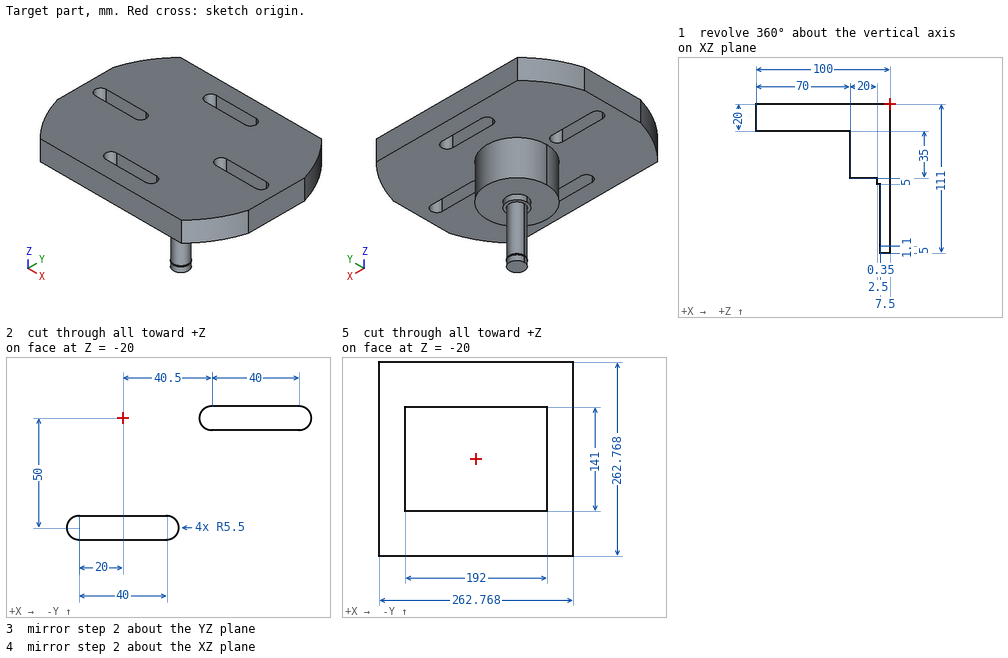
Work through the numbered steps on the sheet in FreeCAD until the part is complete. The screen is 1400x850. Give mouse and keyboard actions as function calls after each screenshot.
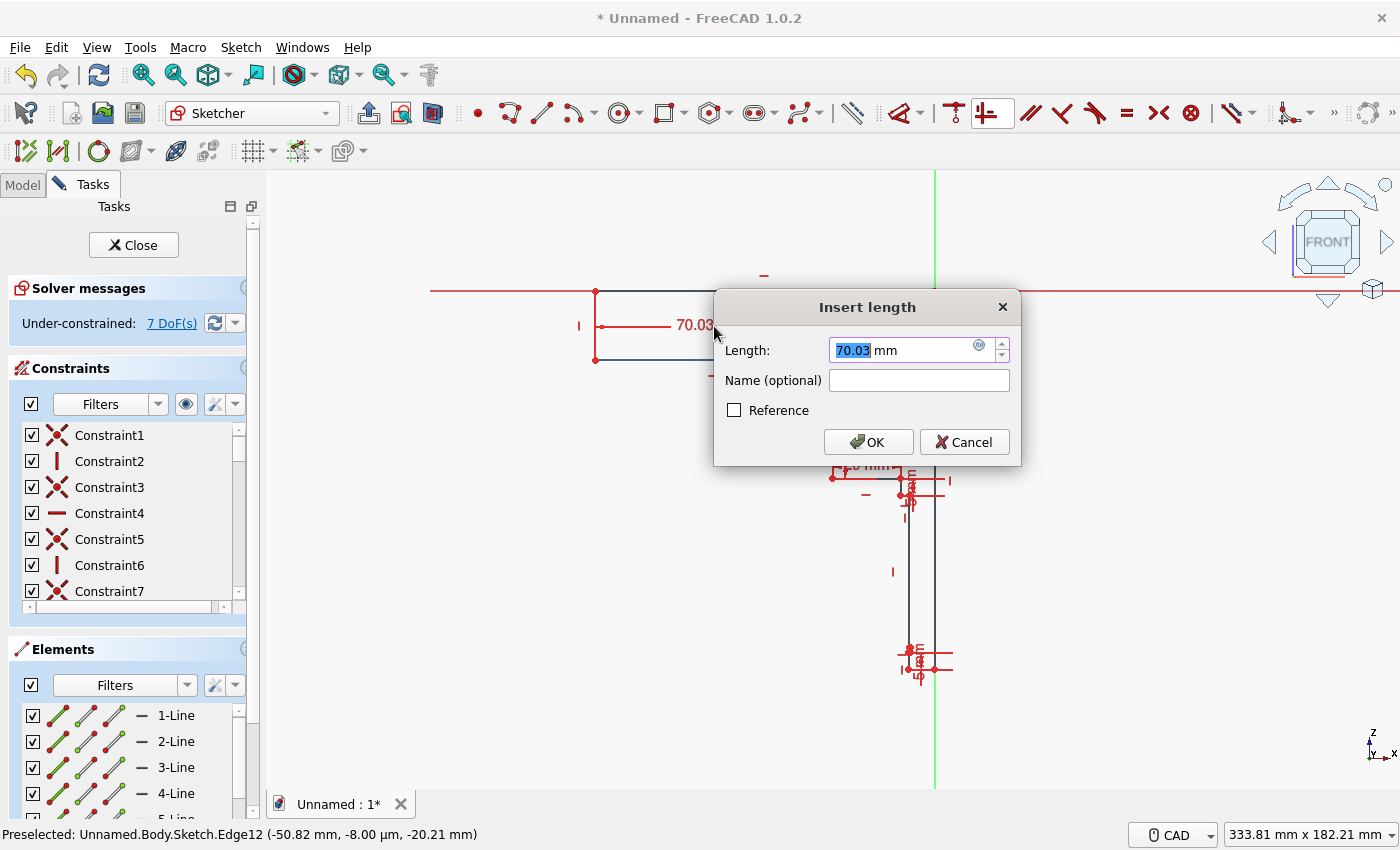
text(70)
key(Return)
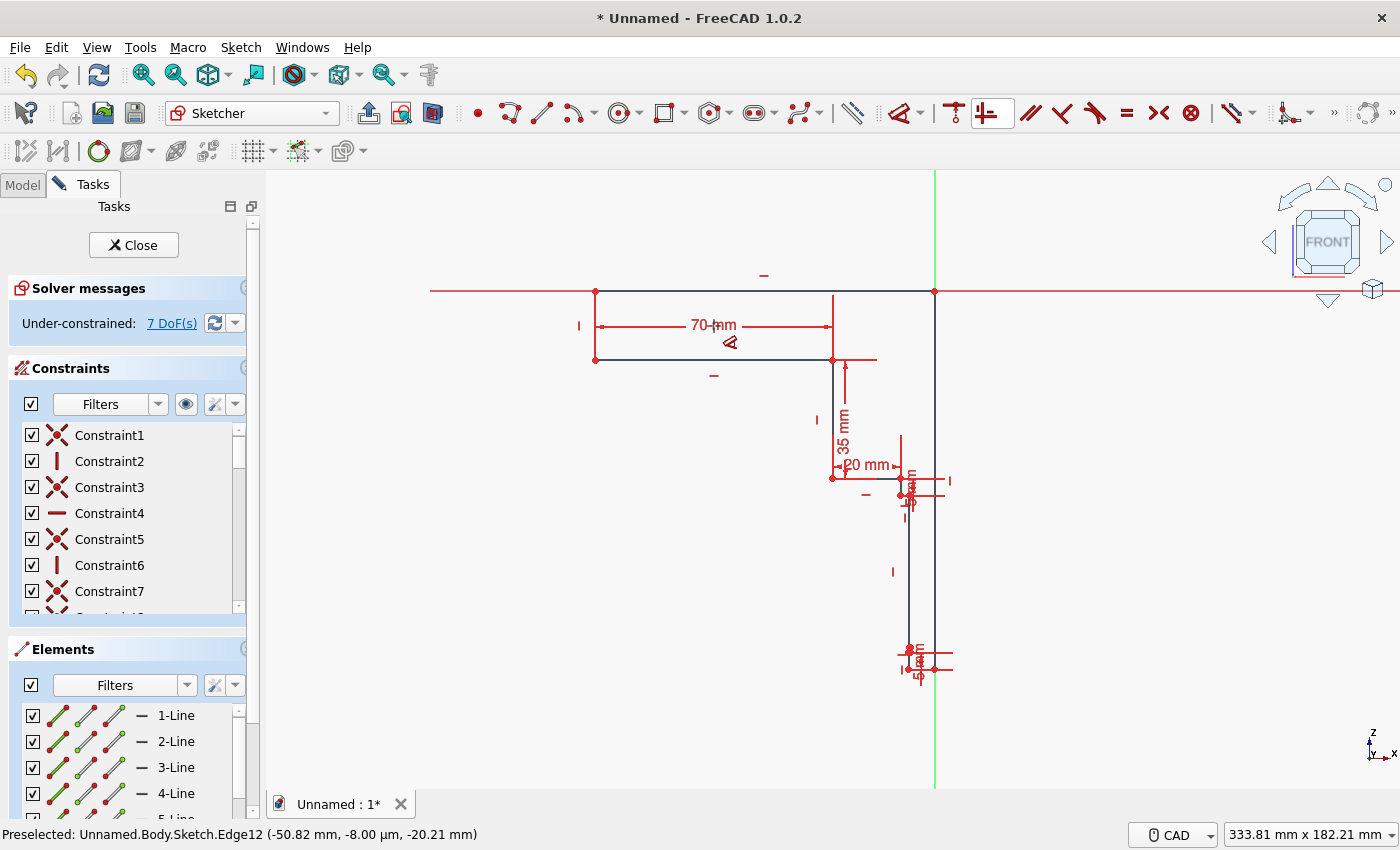
click(595, 339)
click(561, 326)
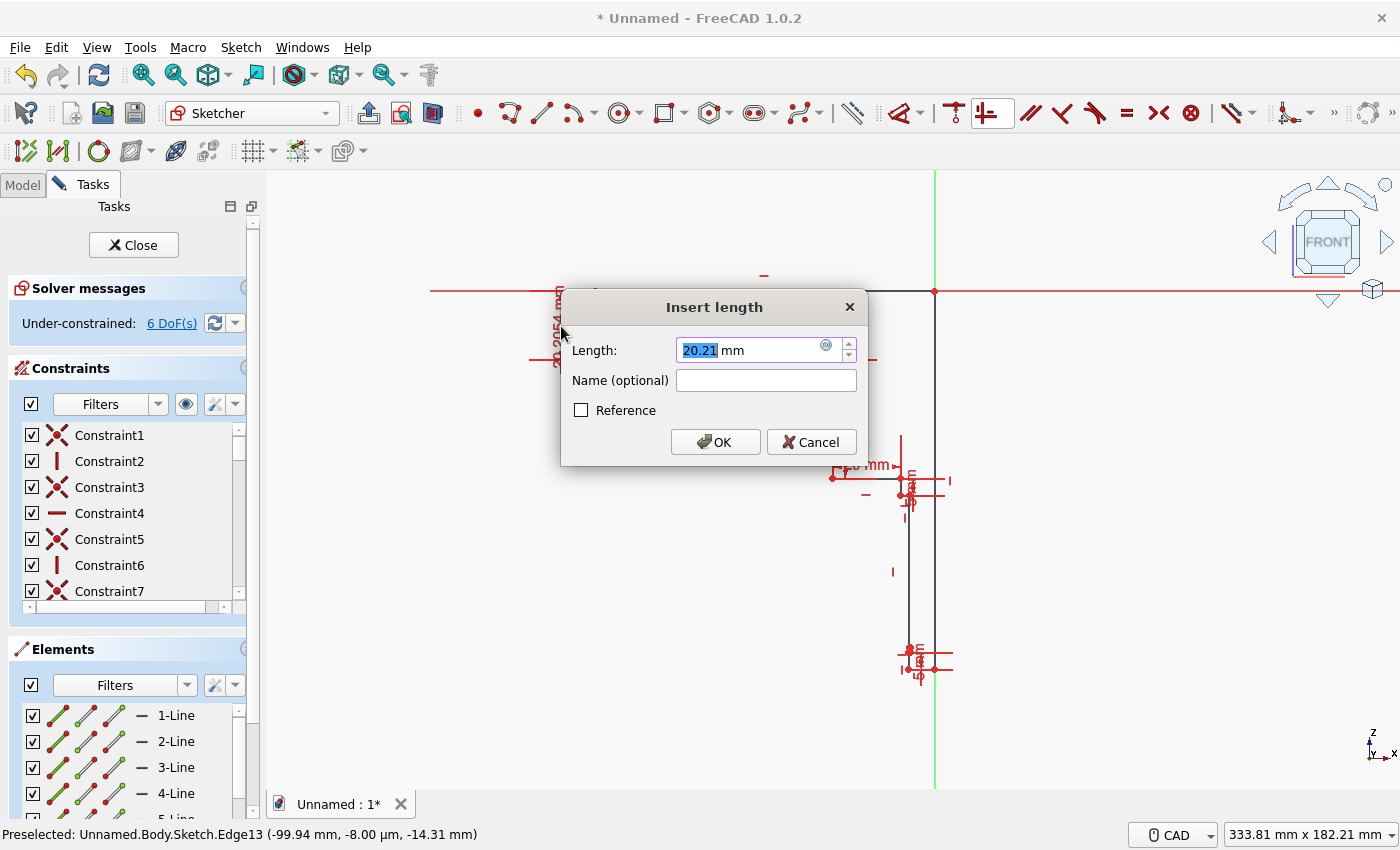
text(20)
key(Return)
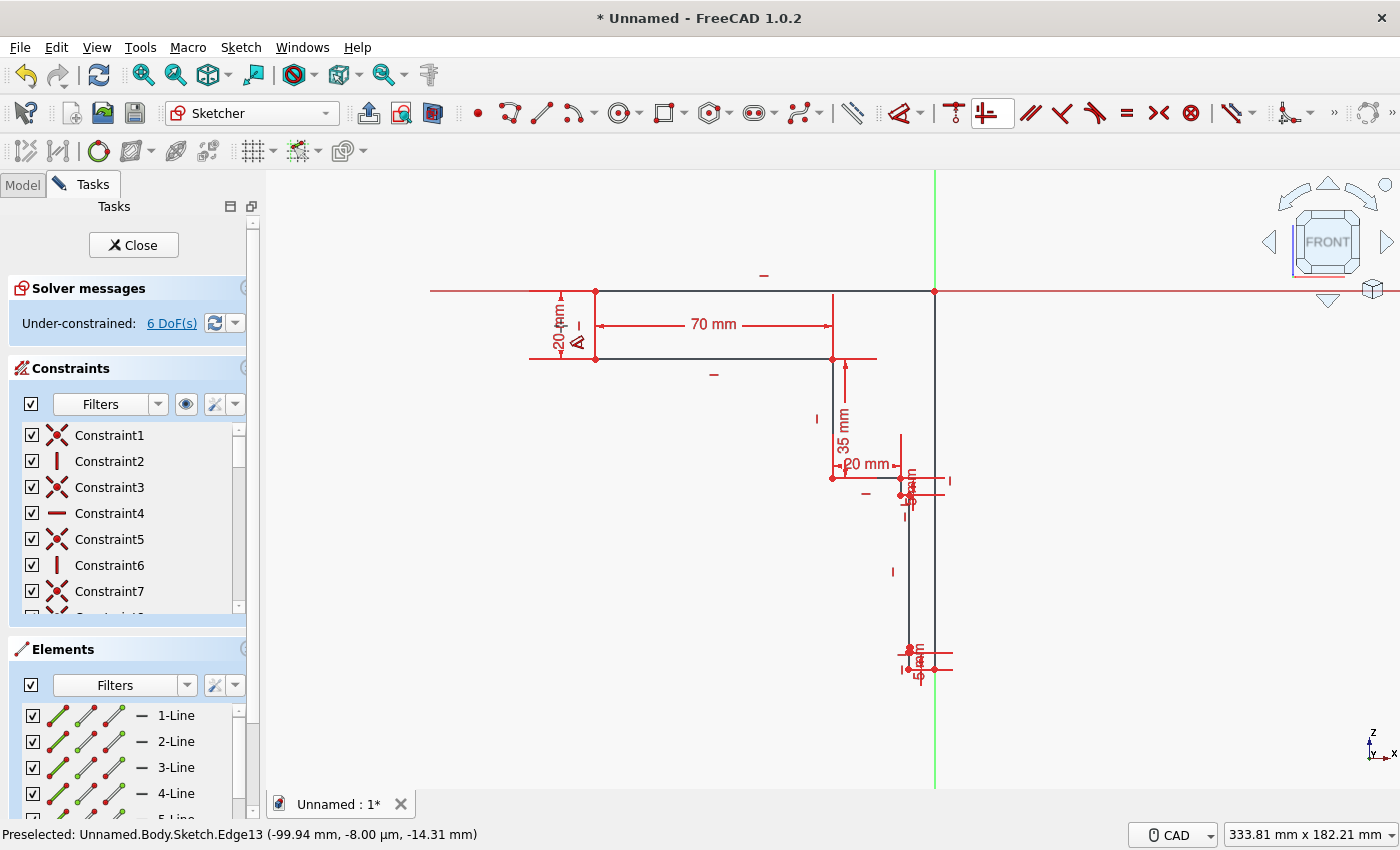
click(935, 405)
click(969, 394)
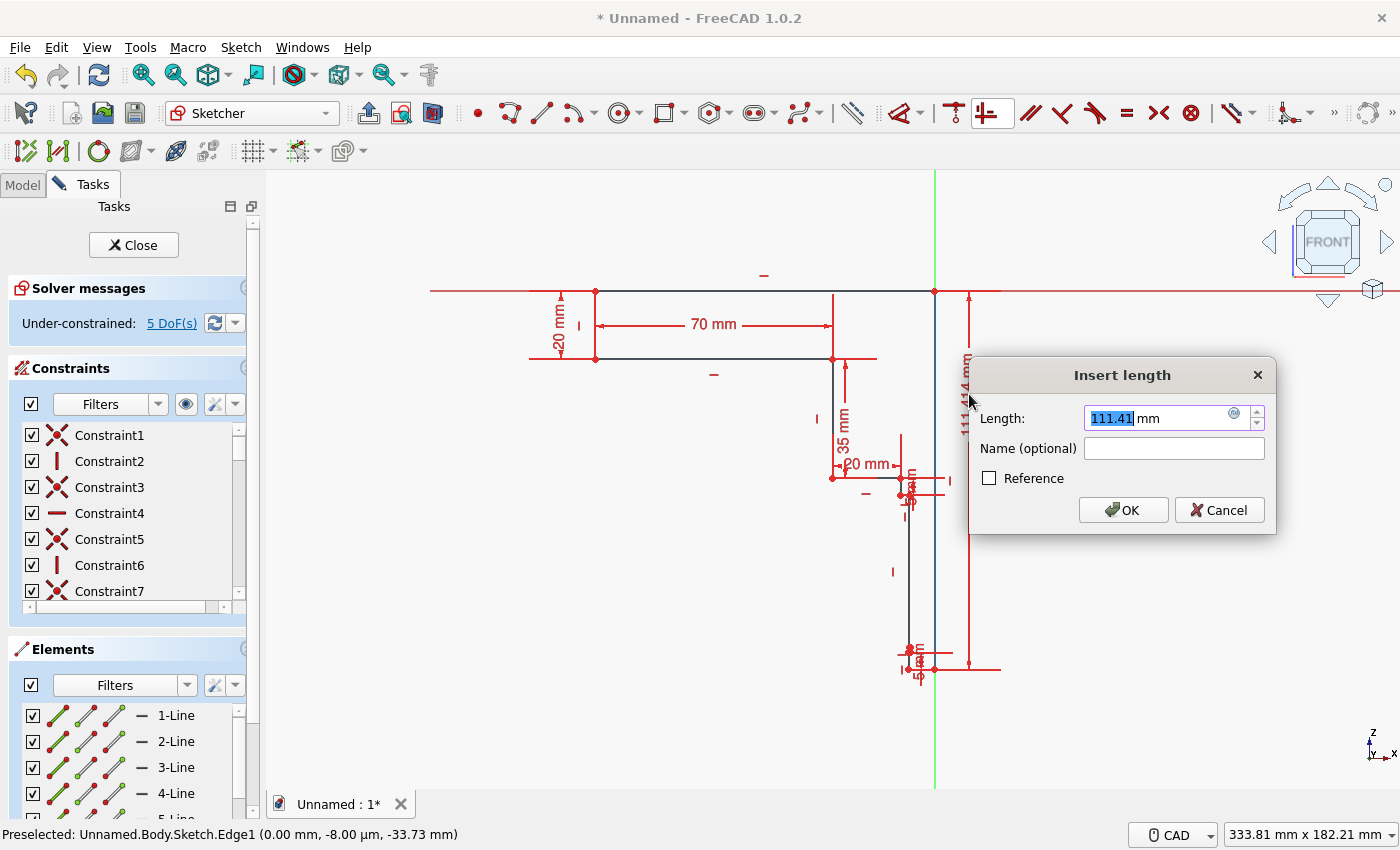
text(111)
key(Return)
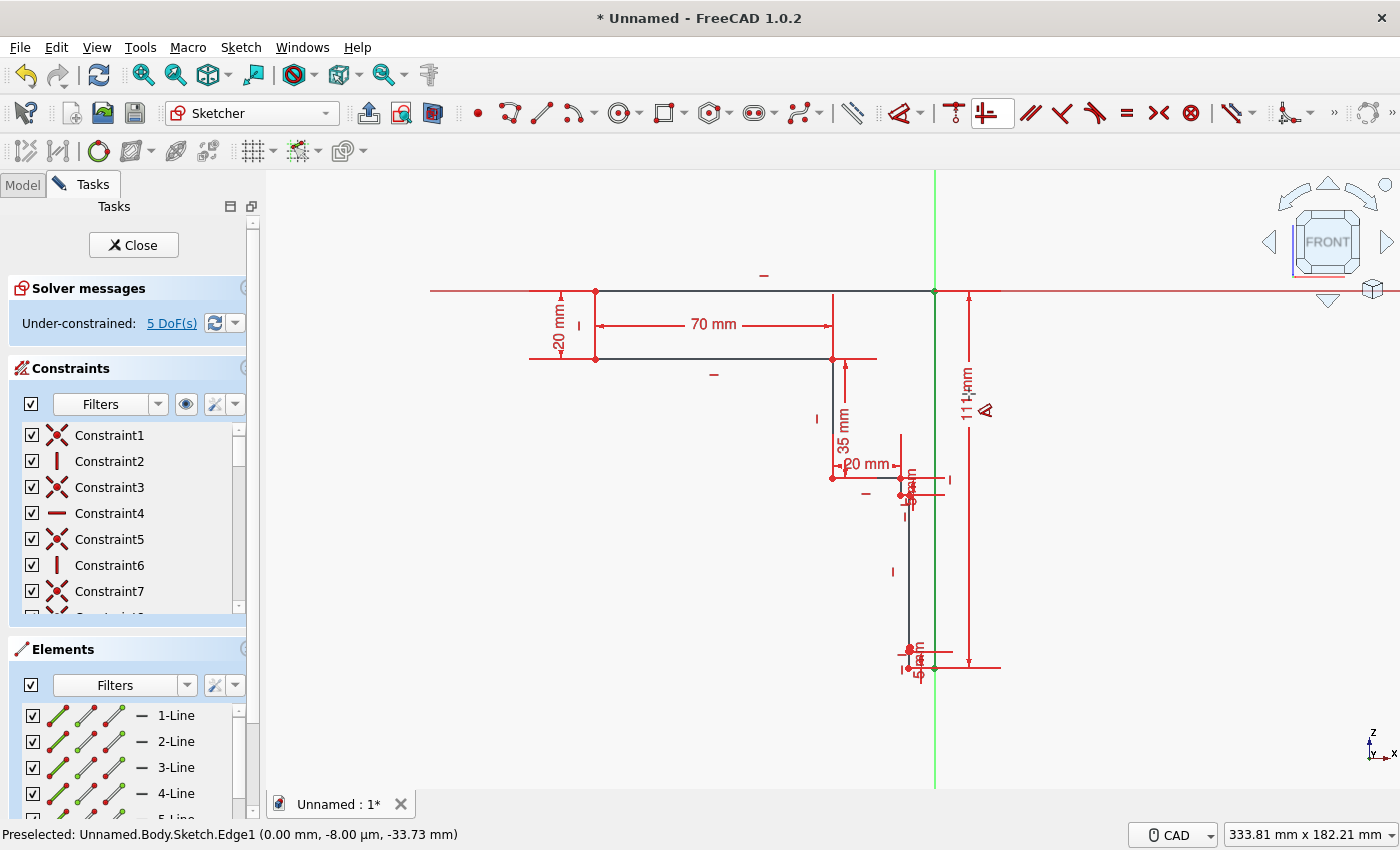
scroll(924, 668, up, 3)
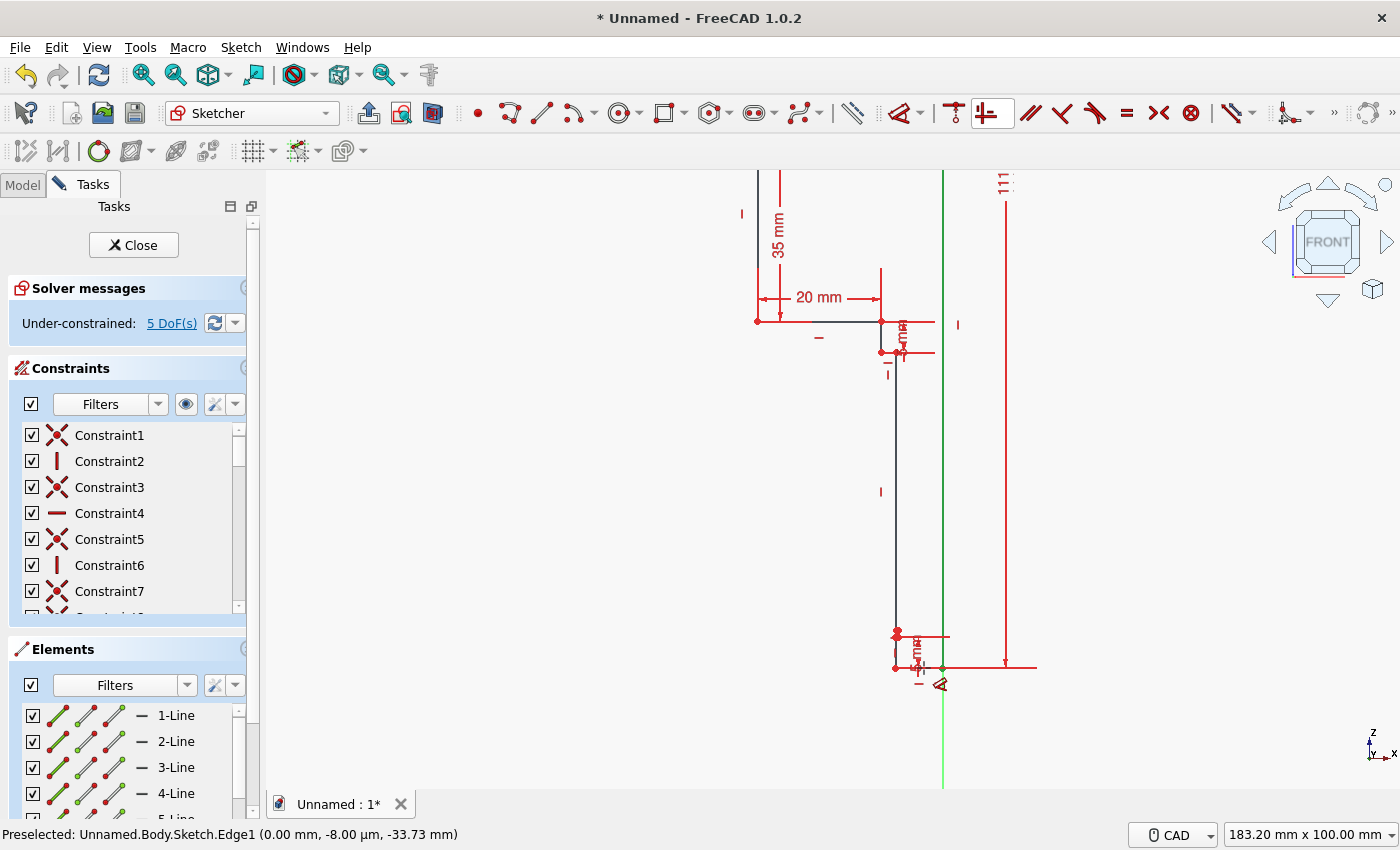
click(924, 668)
click(919, 702)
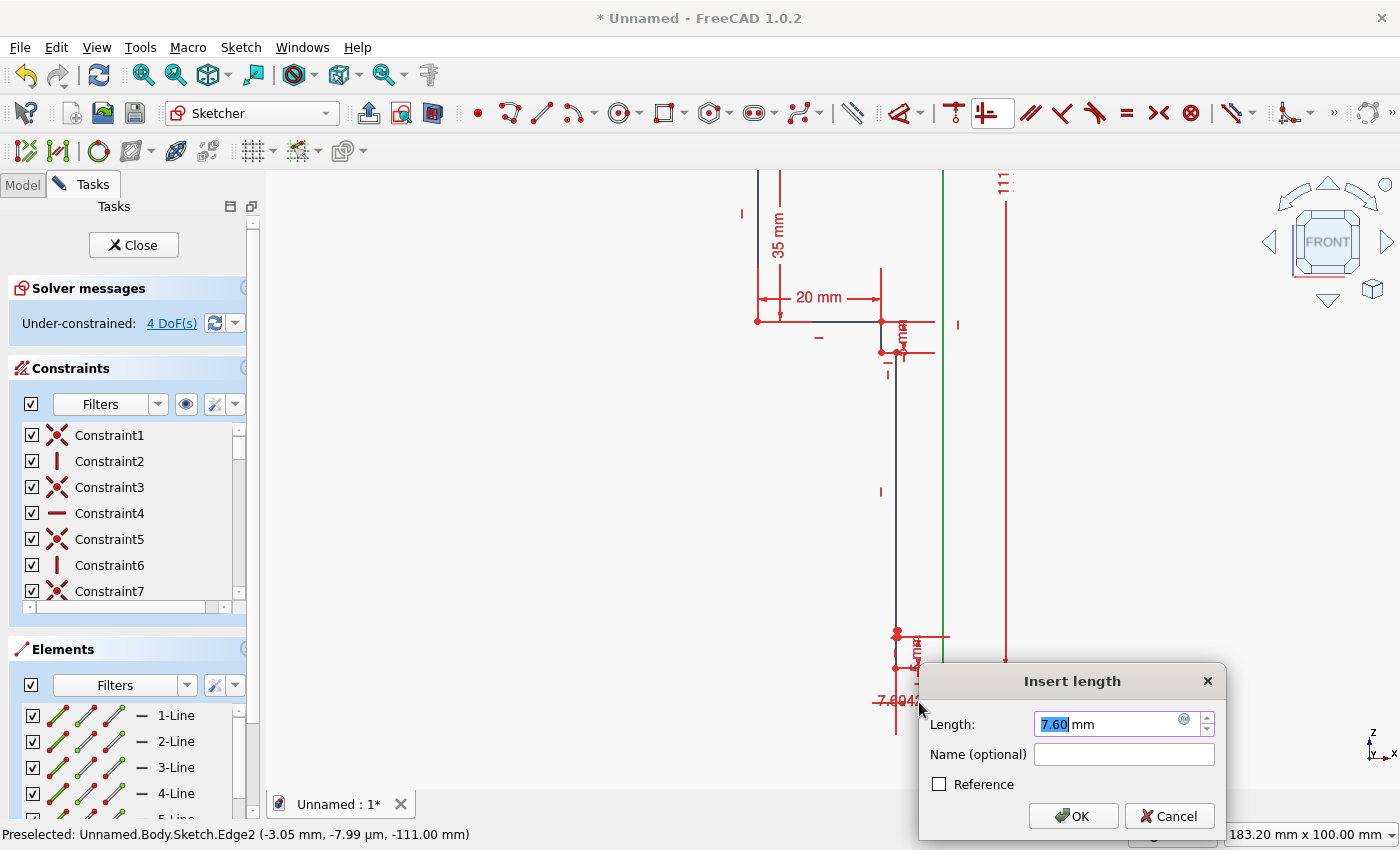
text(7.5)
key(Return)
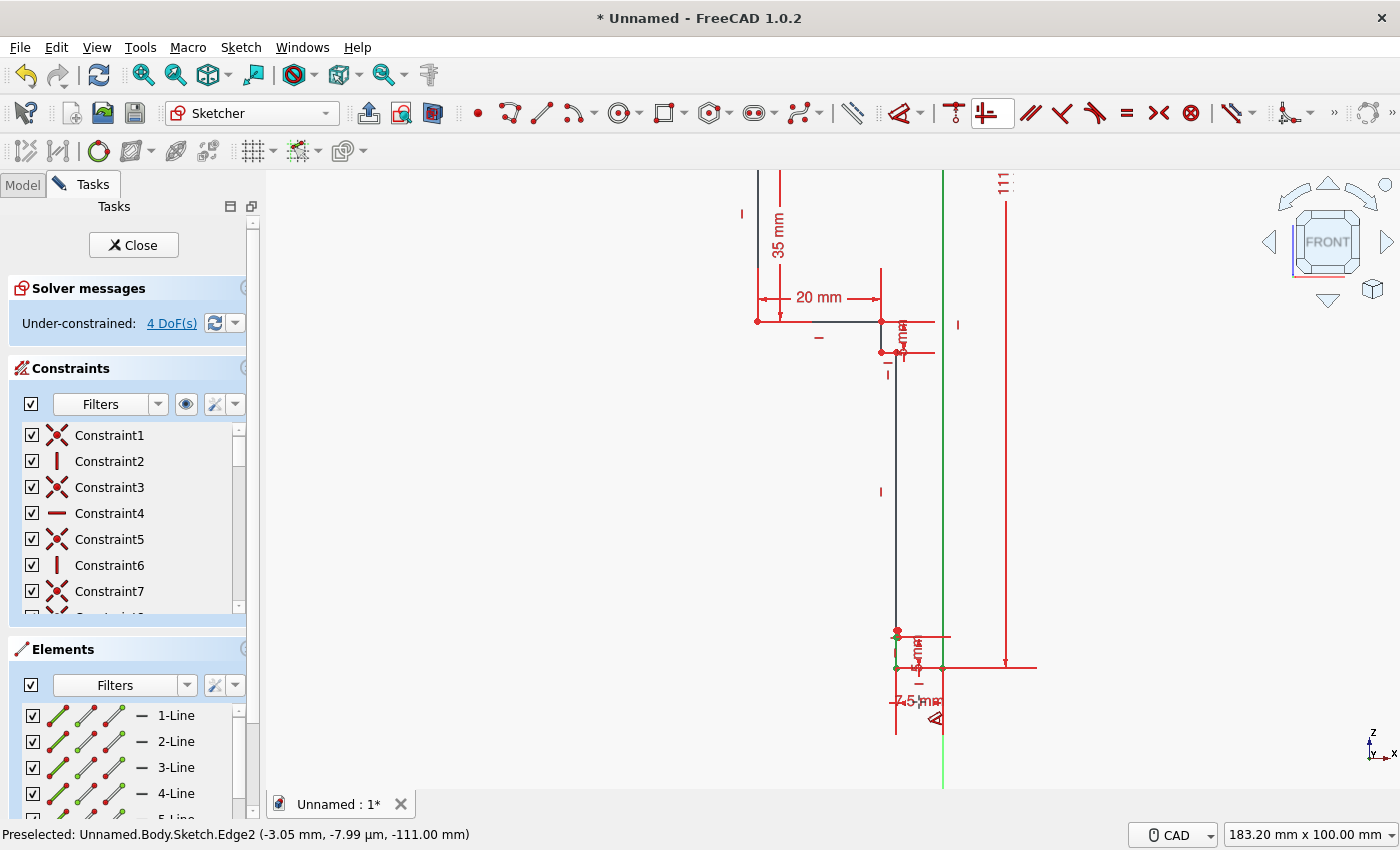
scroll(899, 634, up, 9)